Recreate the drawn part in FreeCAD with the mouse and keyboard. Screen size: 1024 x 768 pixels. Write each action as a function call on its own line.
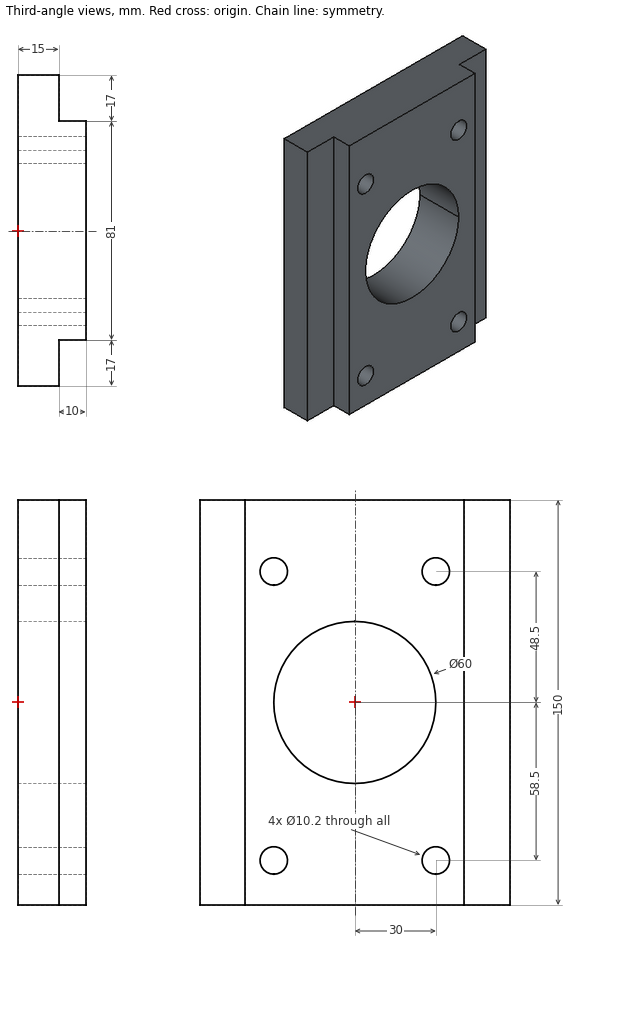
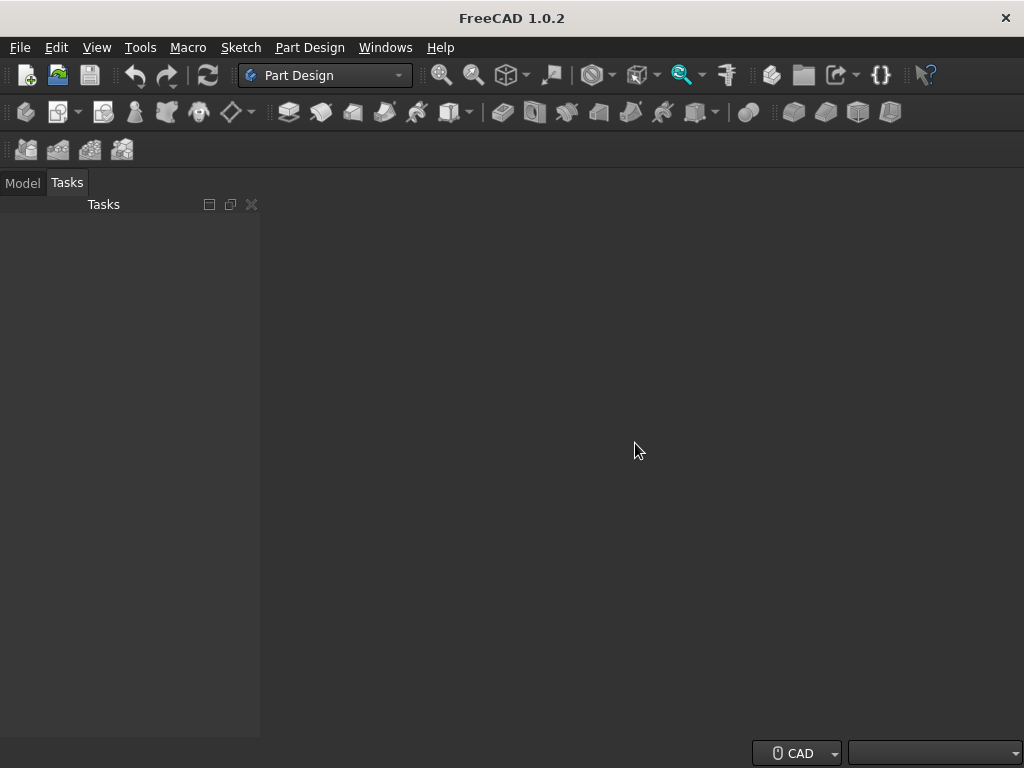
click(26, 76)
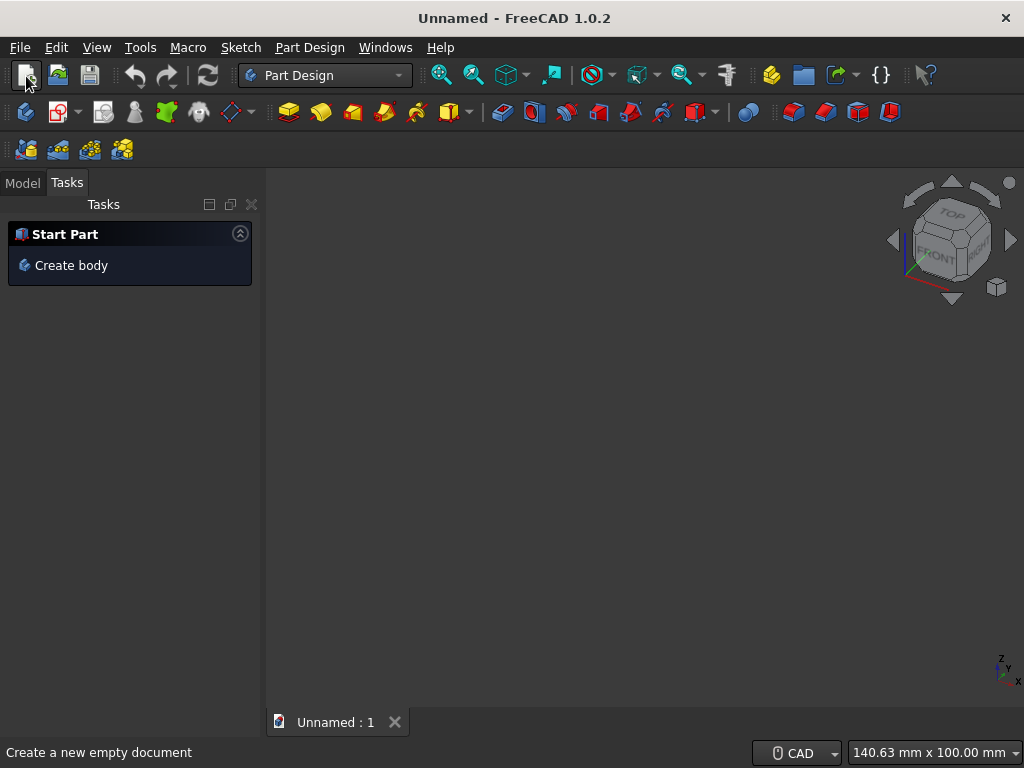
click(58, 112)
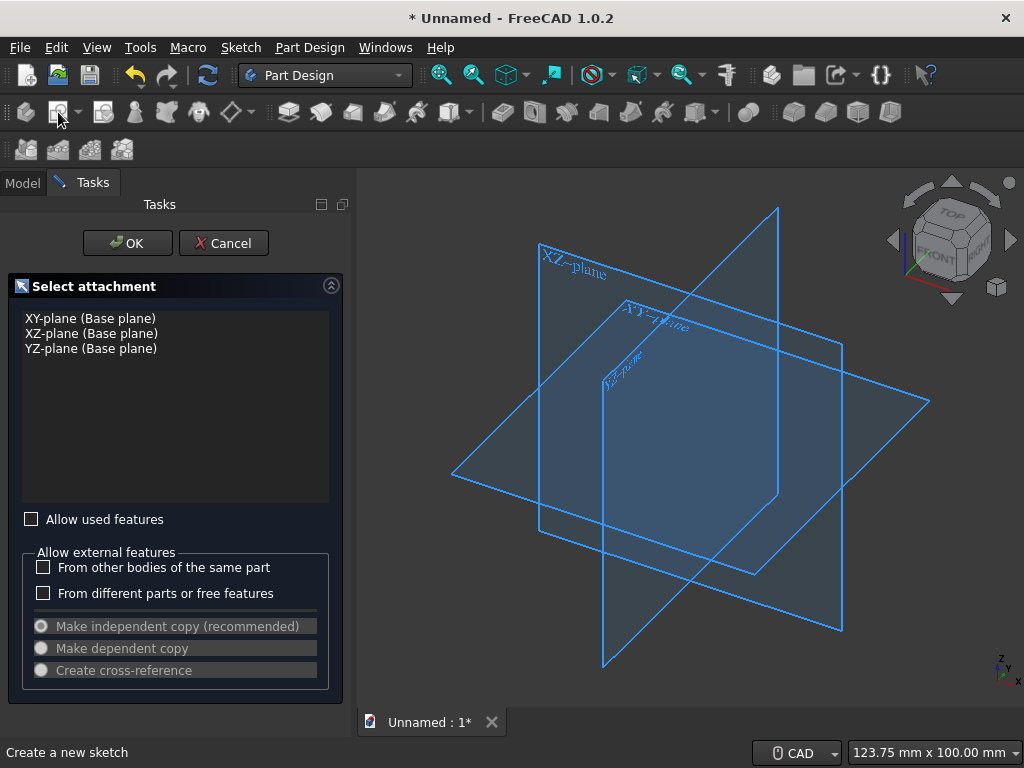
click(82, 318)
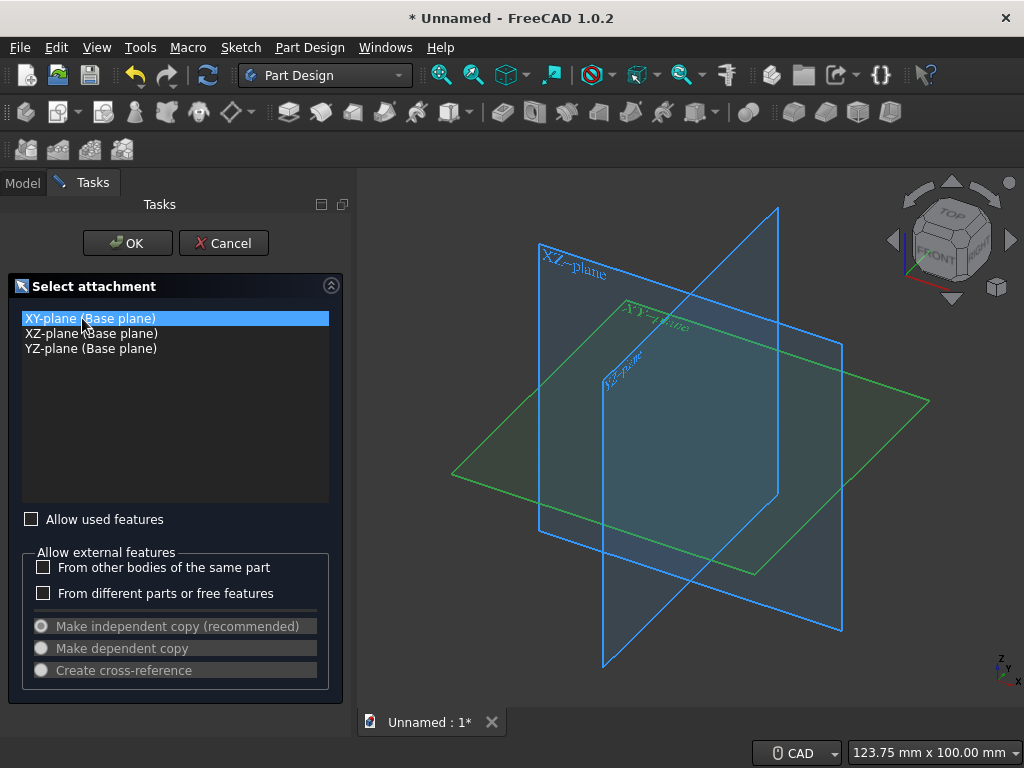
click(128, 243)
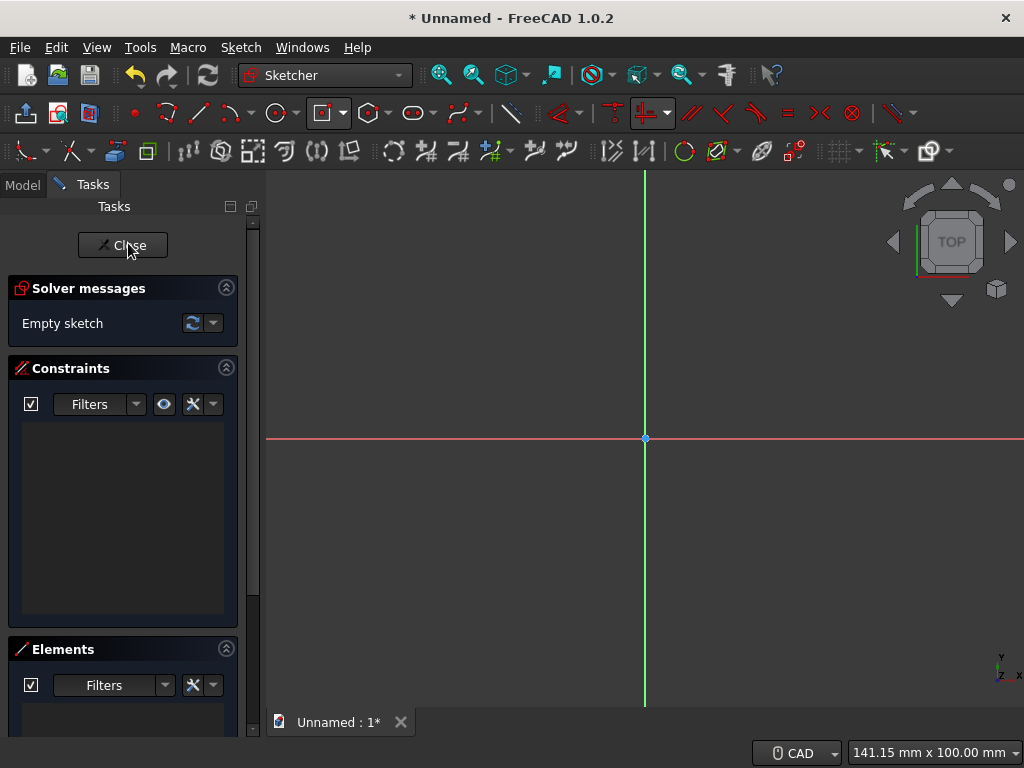
scroll(412, 438, down, 3)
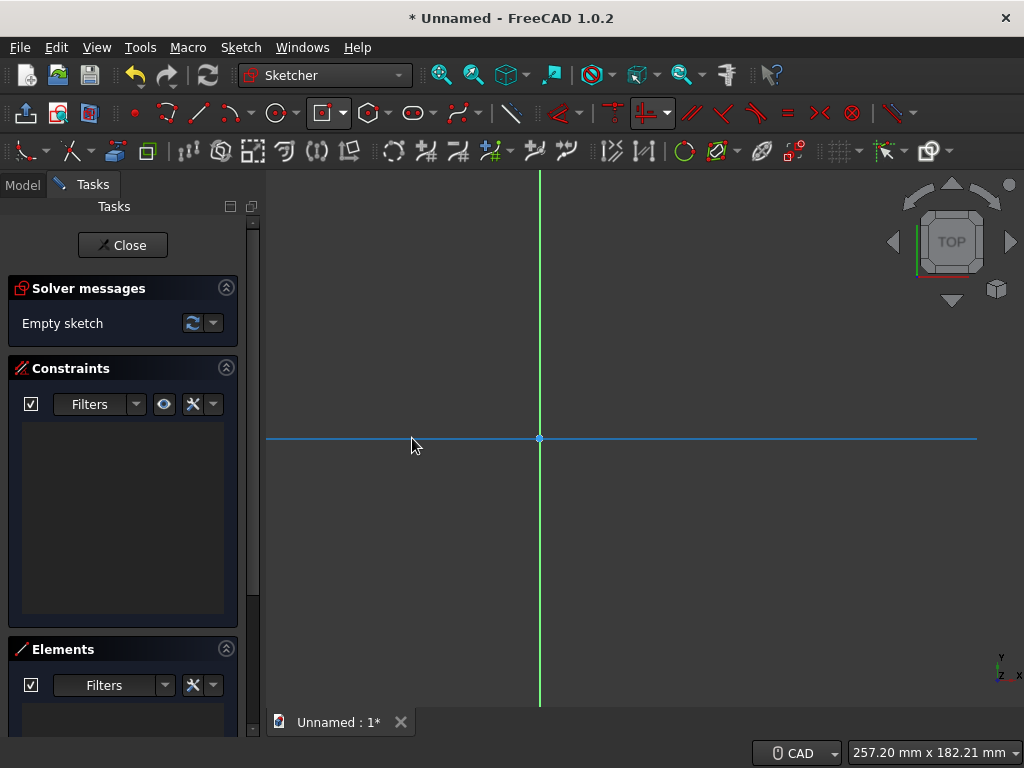
click(168, 114)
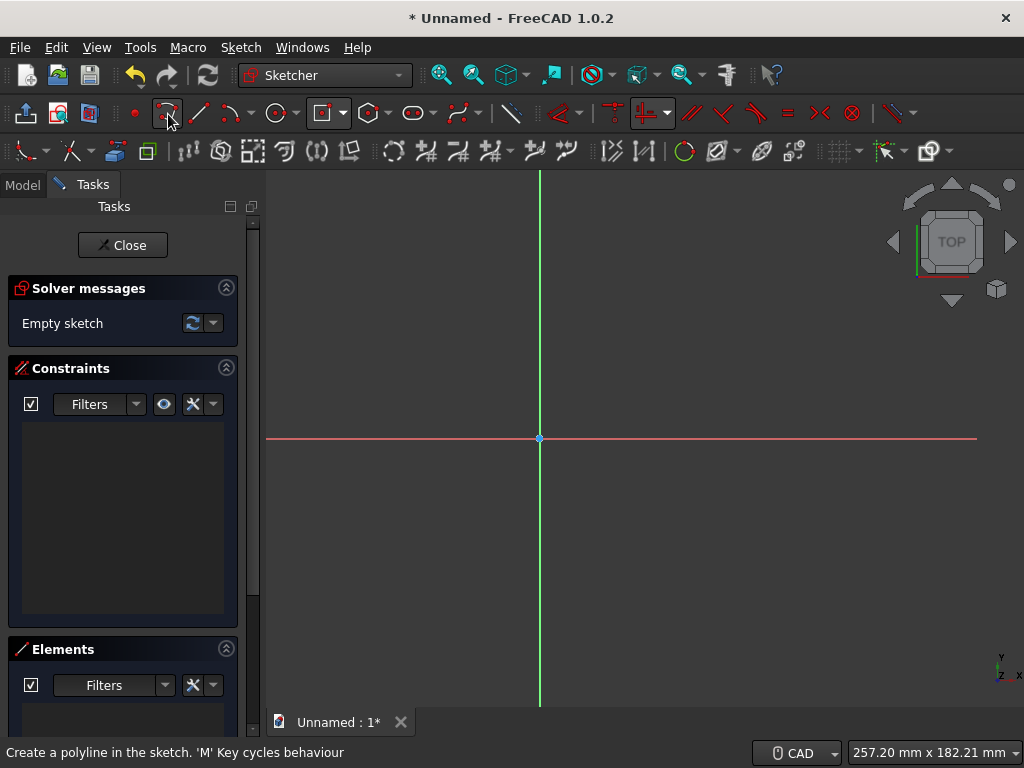
click(584, 558)
click(614, 558)
click(614, 319)
click(584, 319)
click(584, 269)
click(540, 269)
click(549, 608)
click(584, 608)
click(584, 559)
key(Escape)
key(Escape)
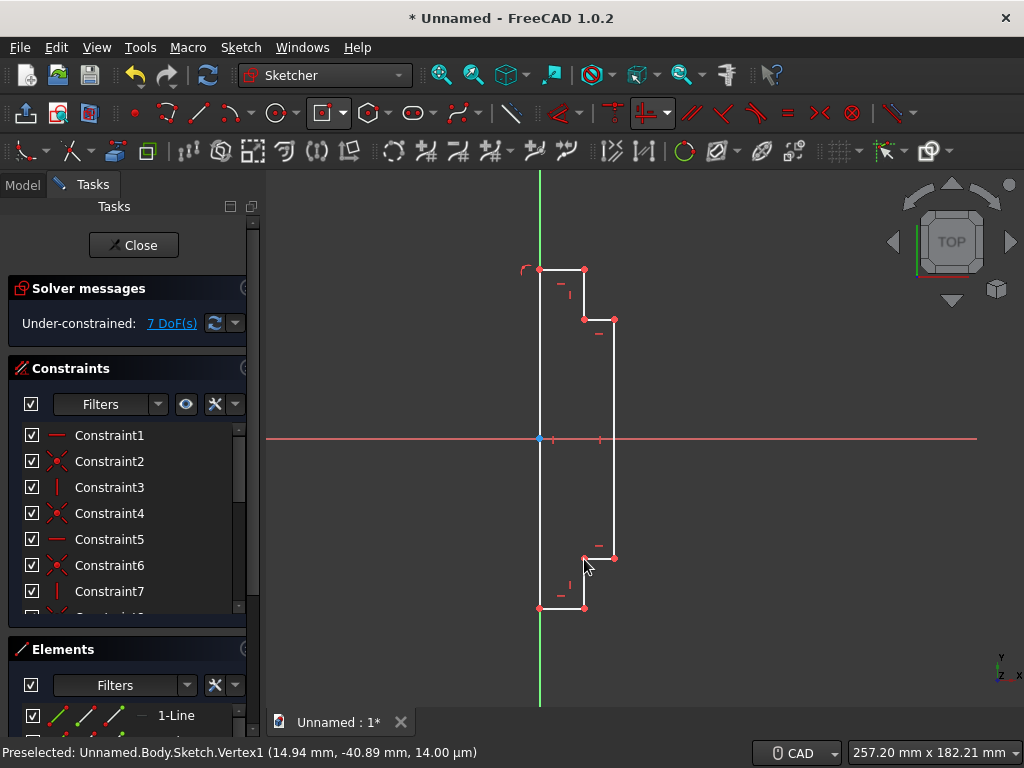
click(584, 559)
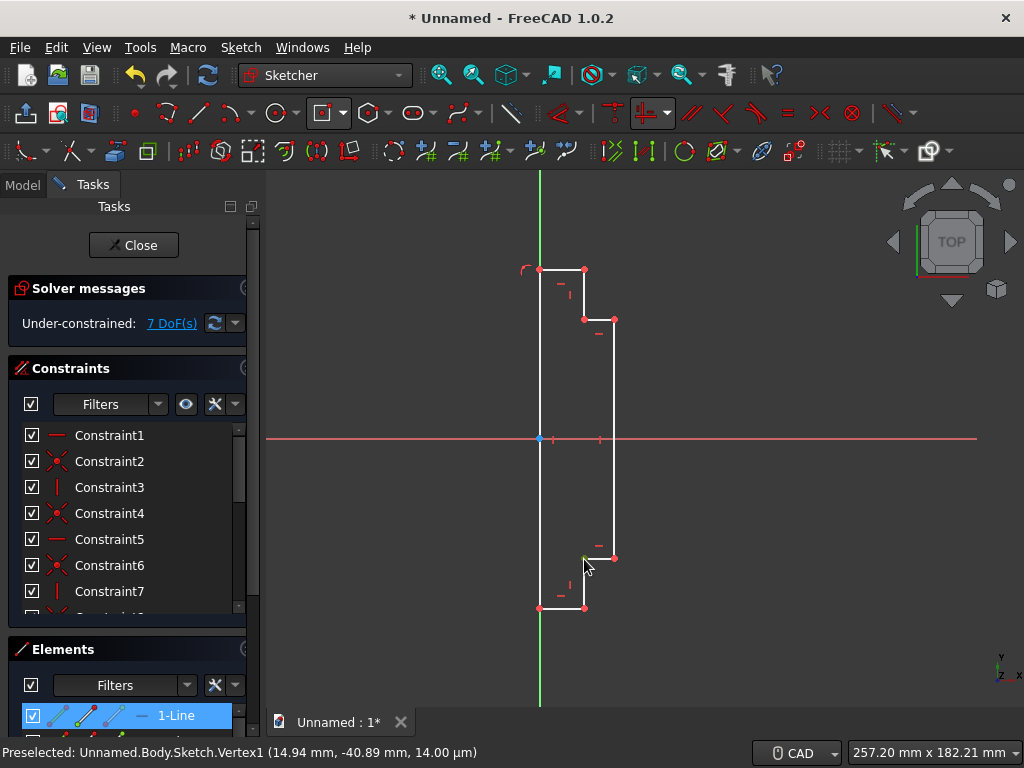
click(584, 320)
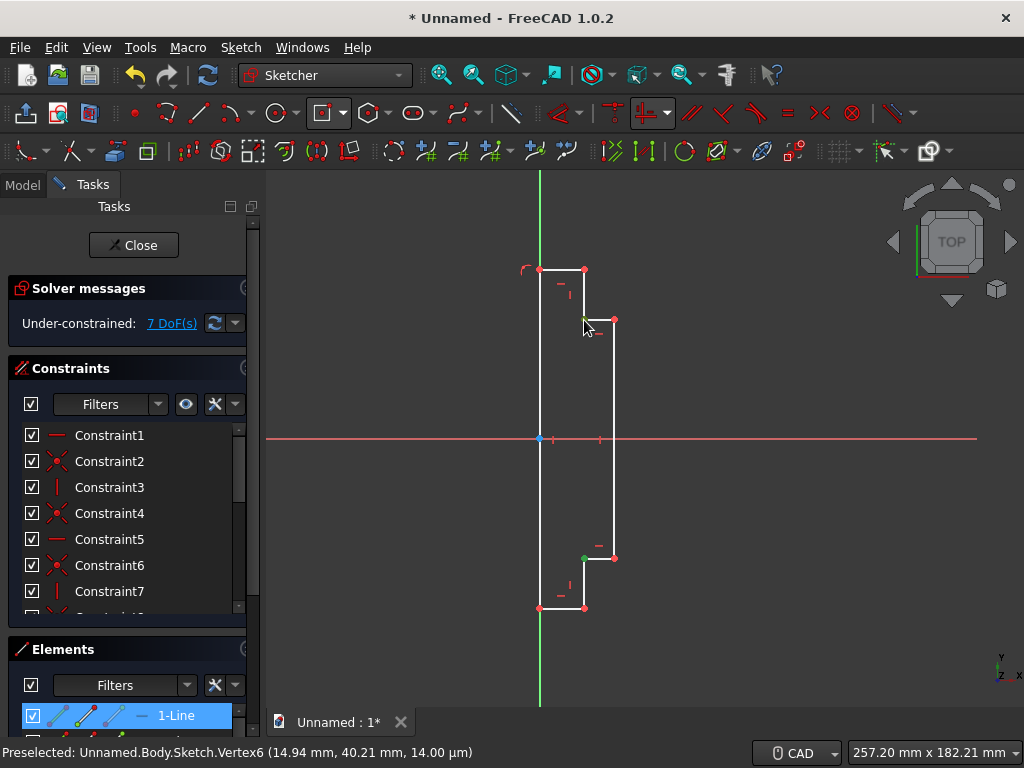
click(334, 438)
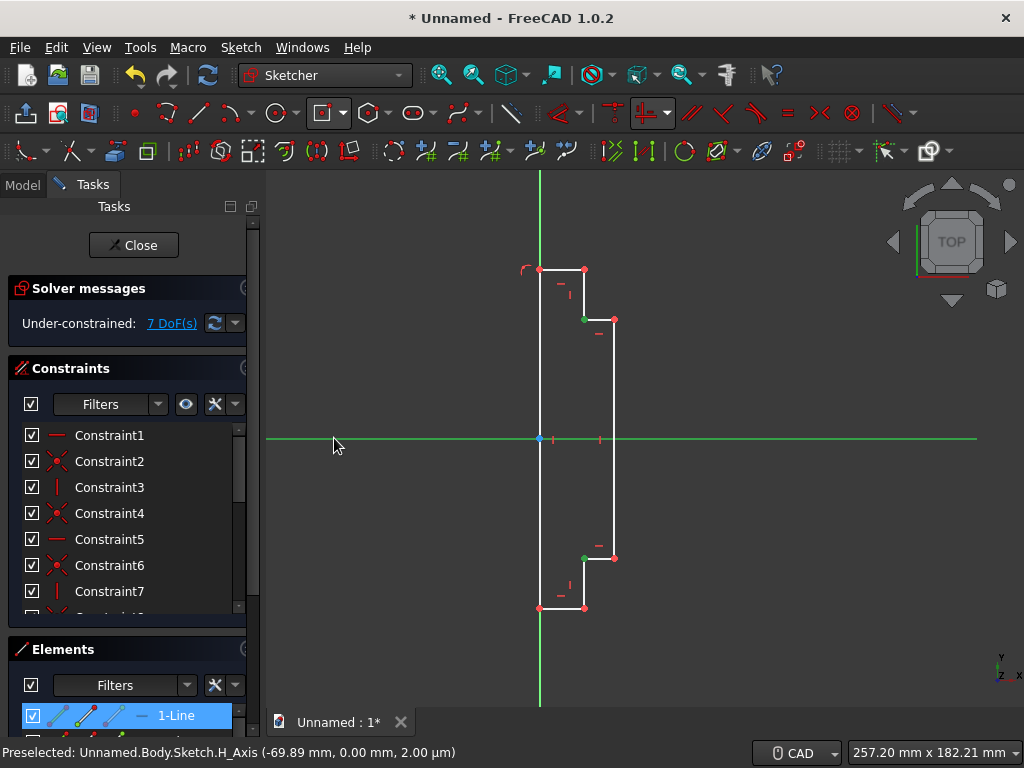
click(820, 114)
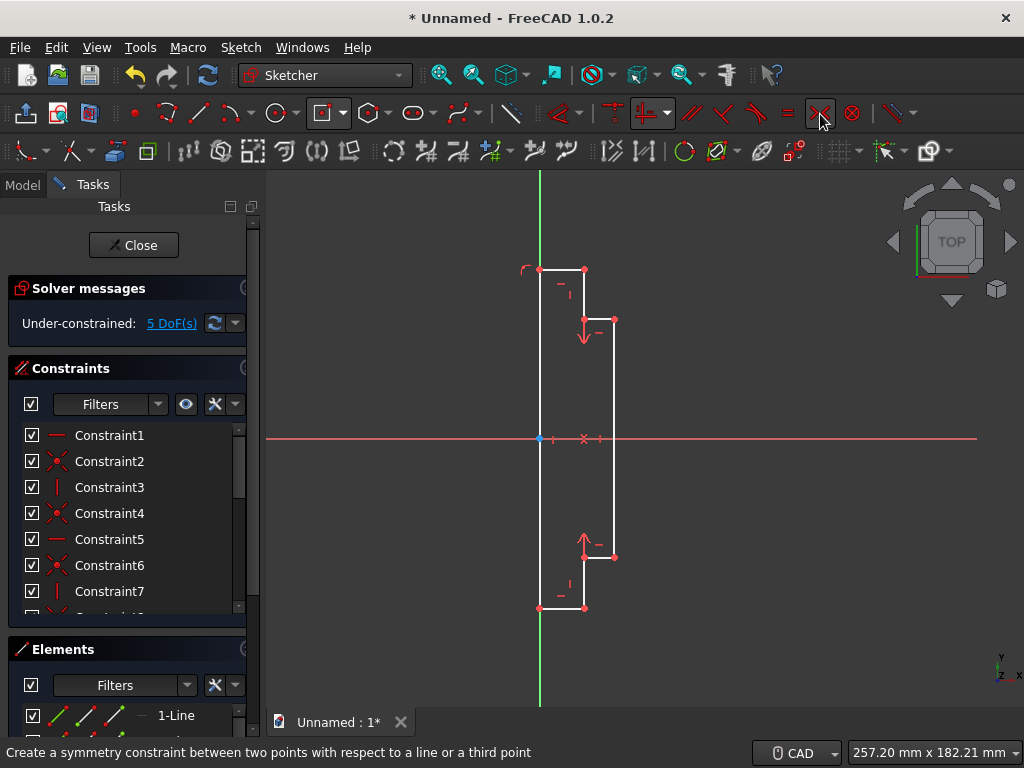
click(558, 114)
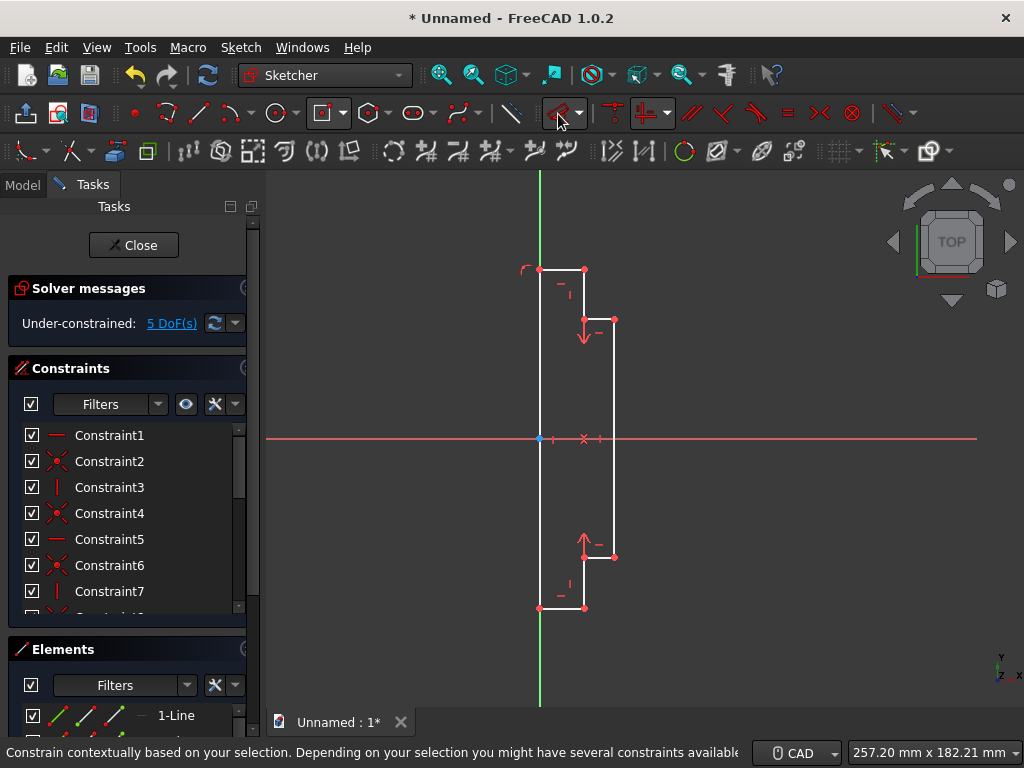
scroll(593, 558, up, 3)